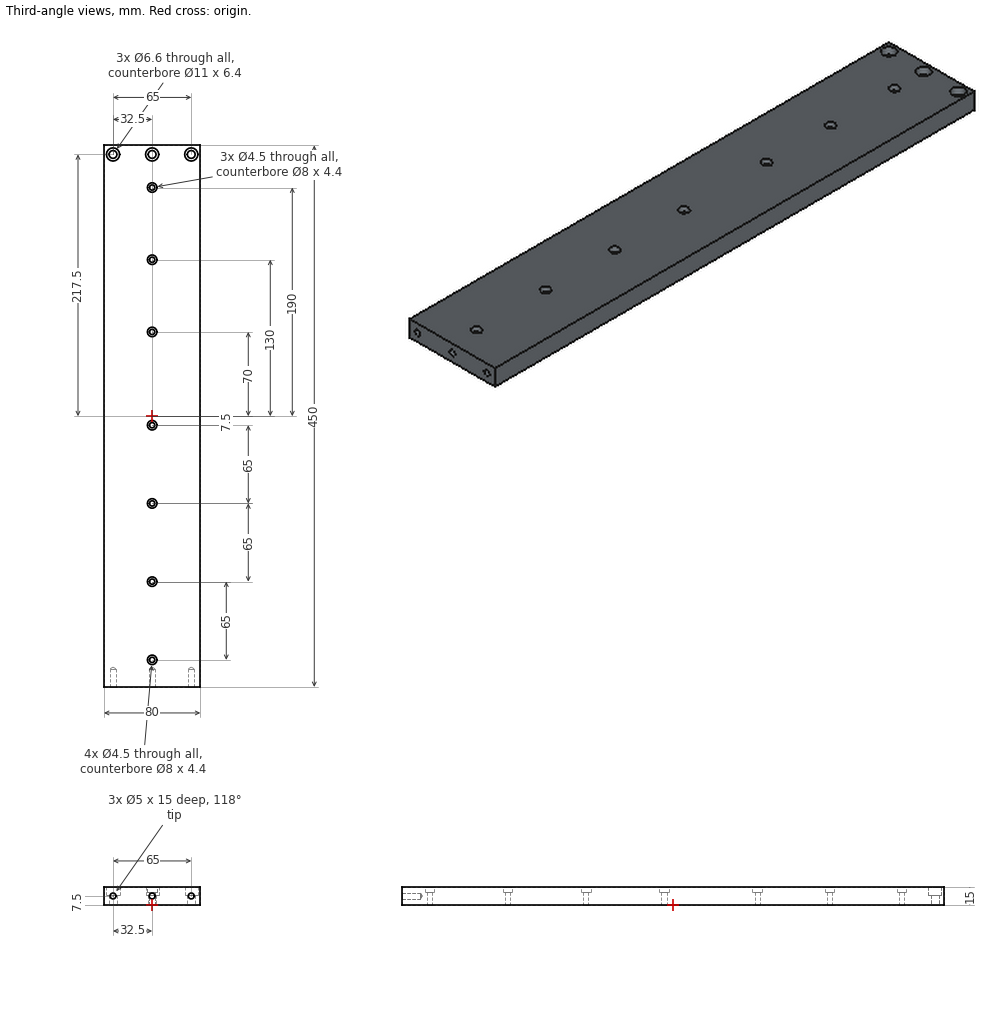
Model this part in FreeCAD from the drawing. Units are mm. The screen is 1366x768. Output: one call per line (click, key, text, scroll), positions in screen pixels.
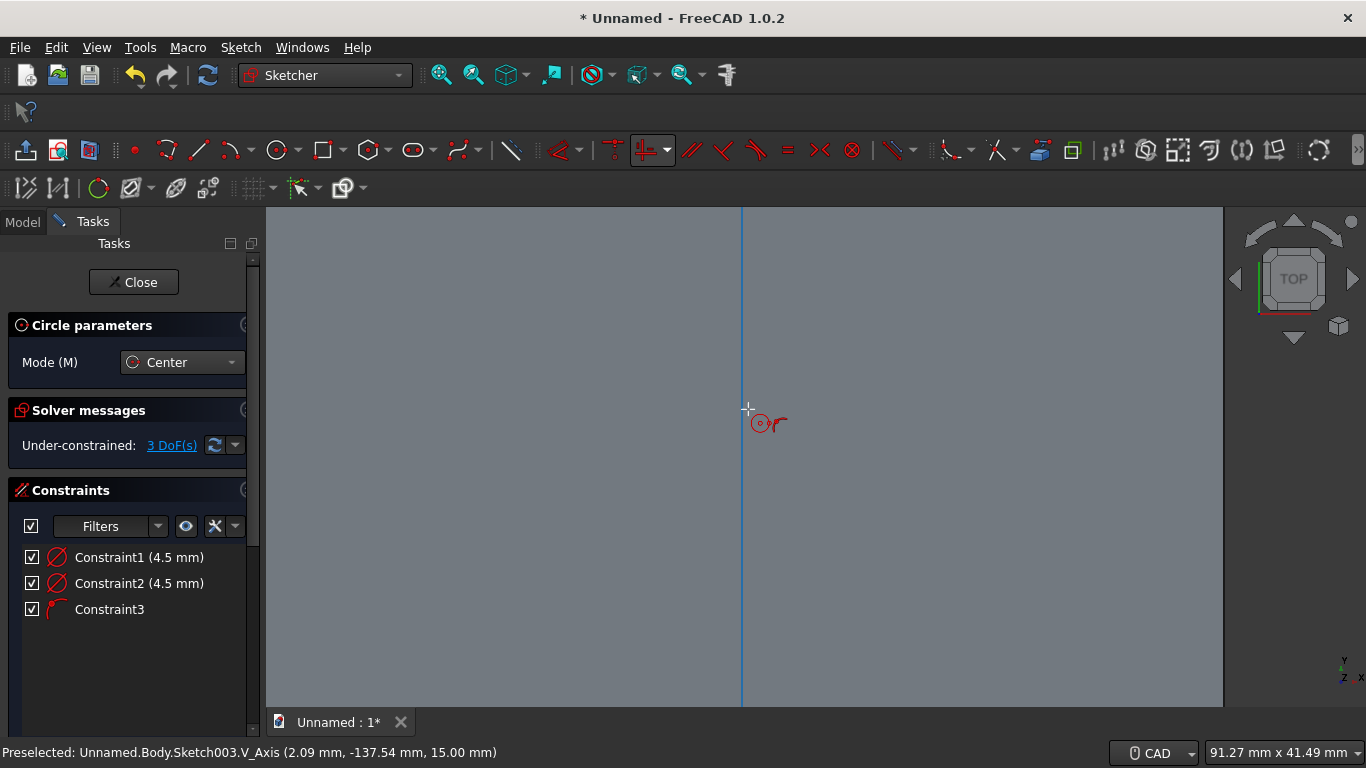
scroll(748, 409, down, 10)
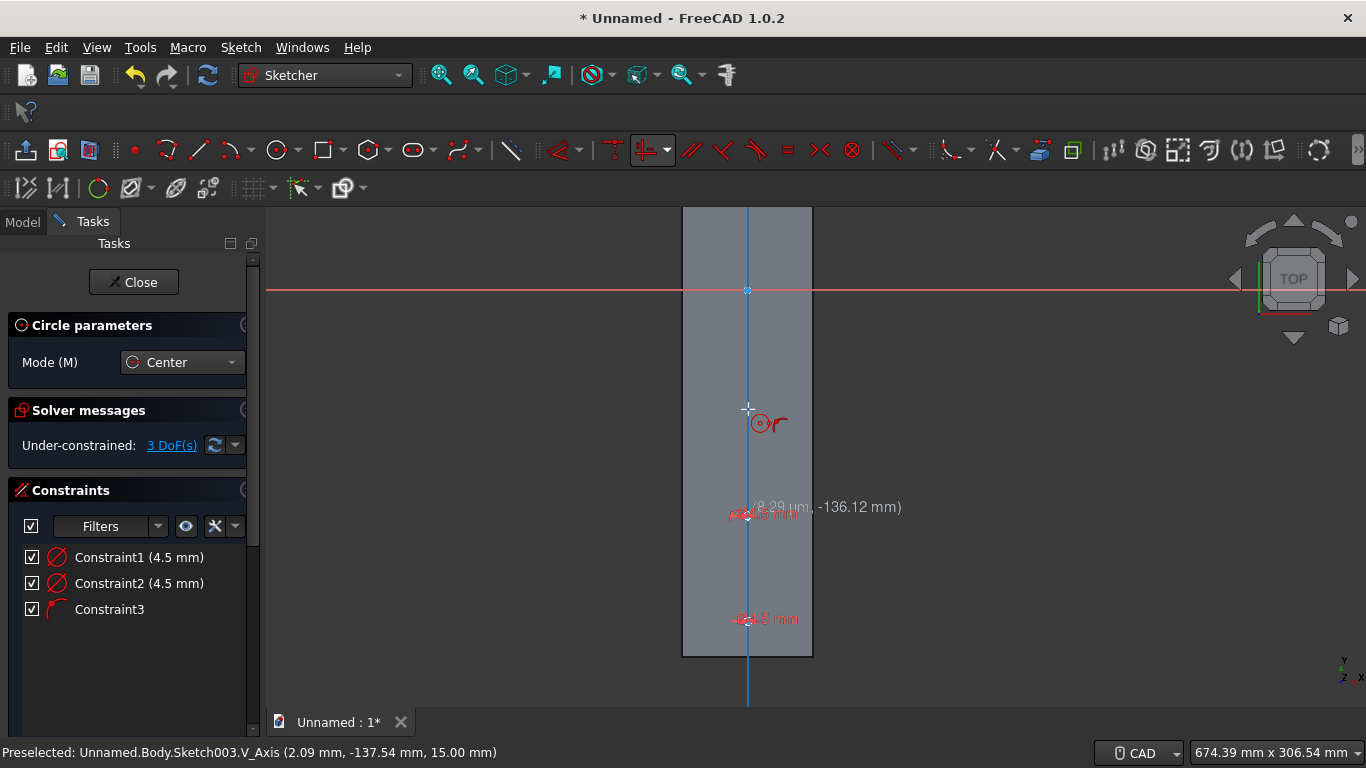
click(748, 409)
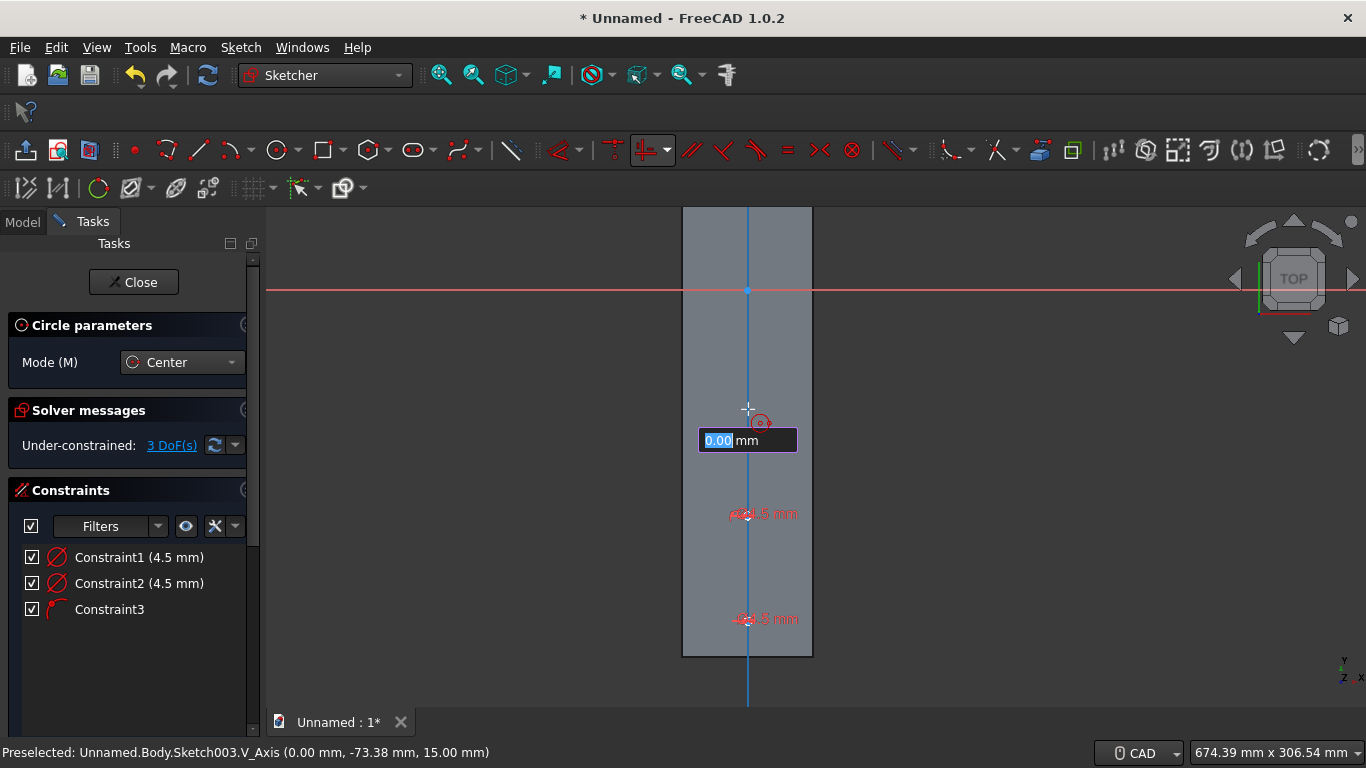
scroll(751, 407, up, 8)
move(750, 407)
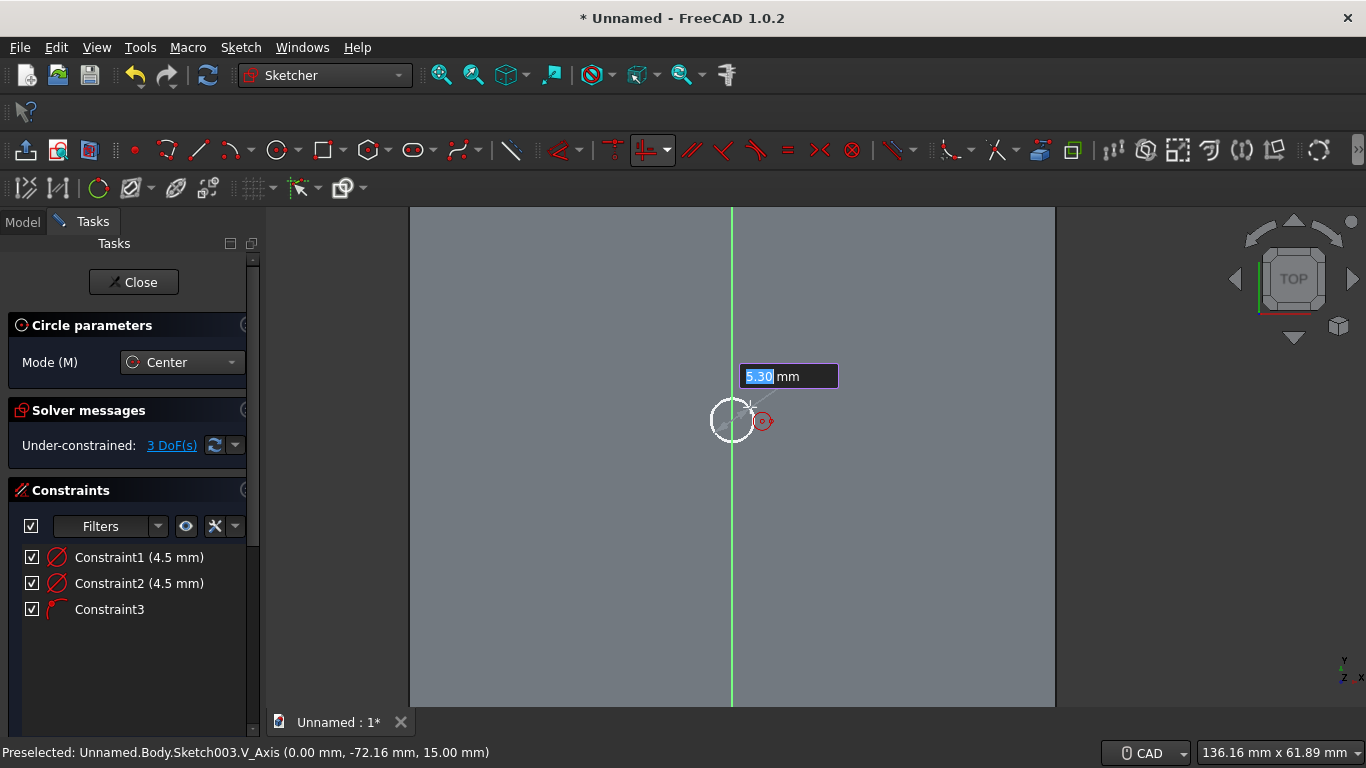
text(4.5)
key(Return)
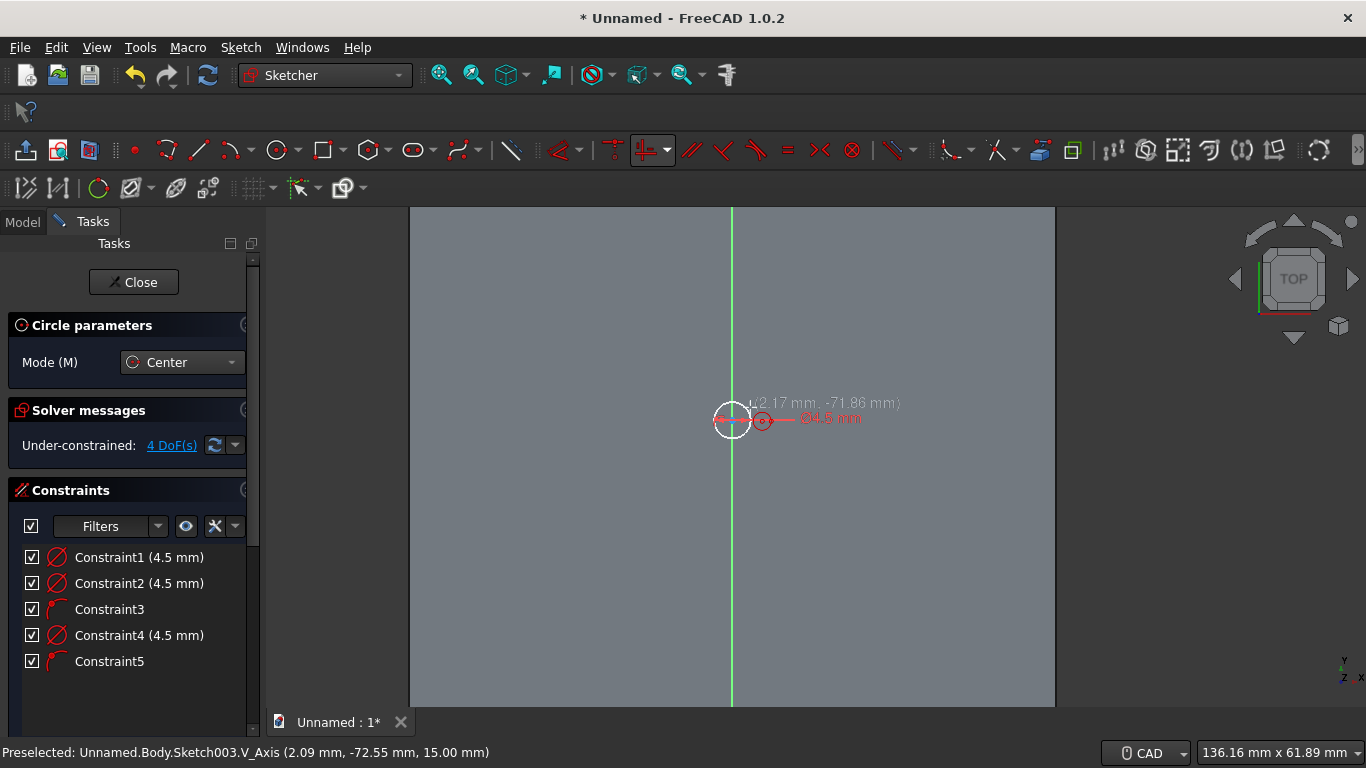
scroll(751, 407, down, 8)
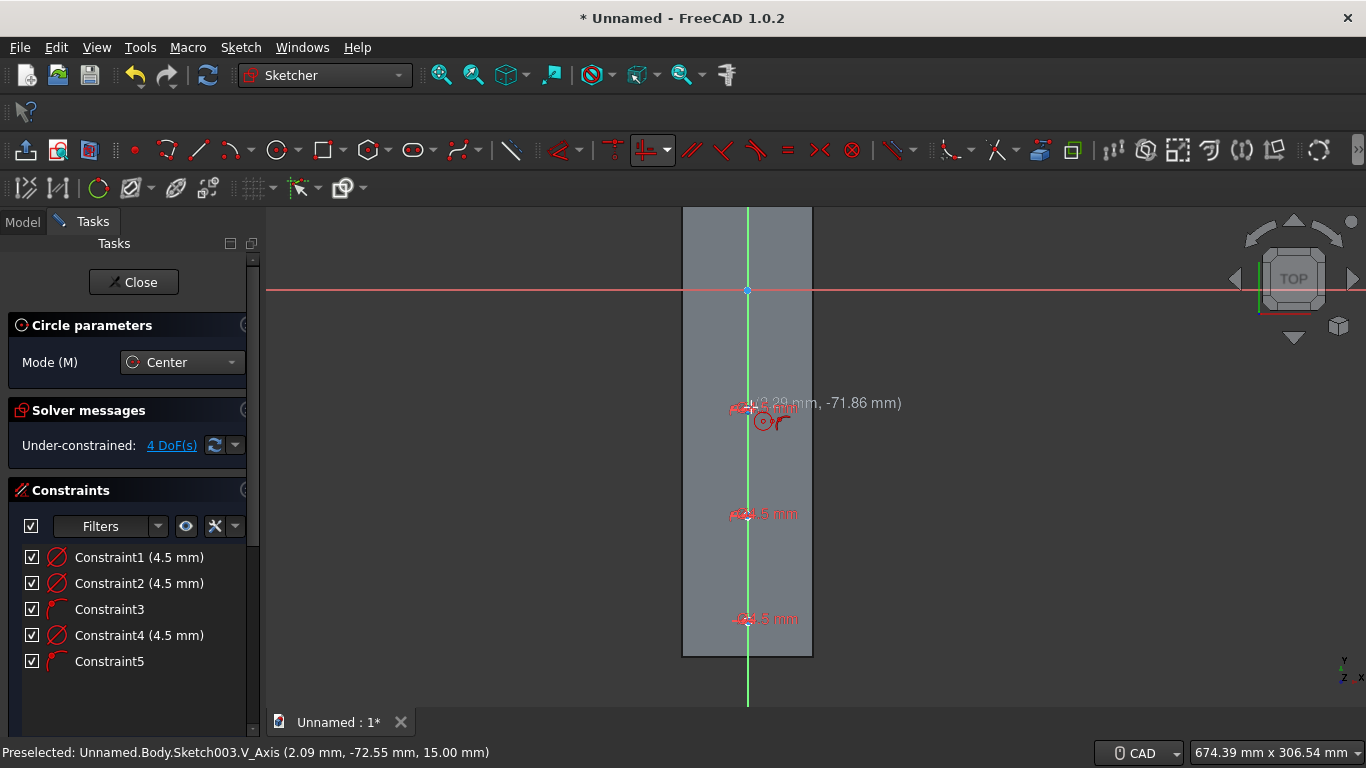
scroll(748, 303, up, 10)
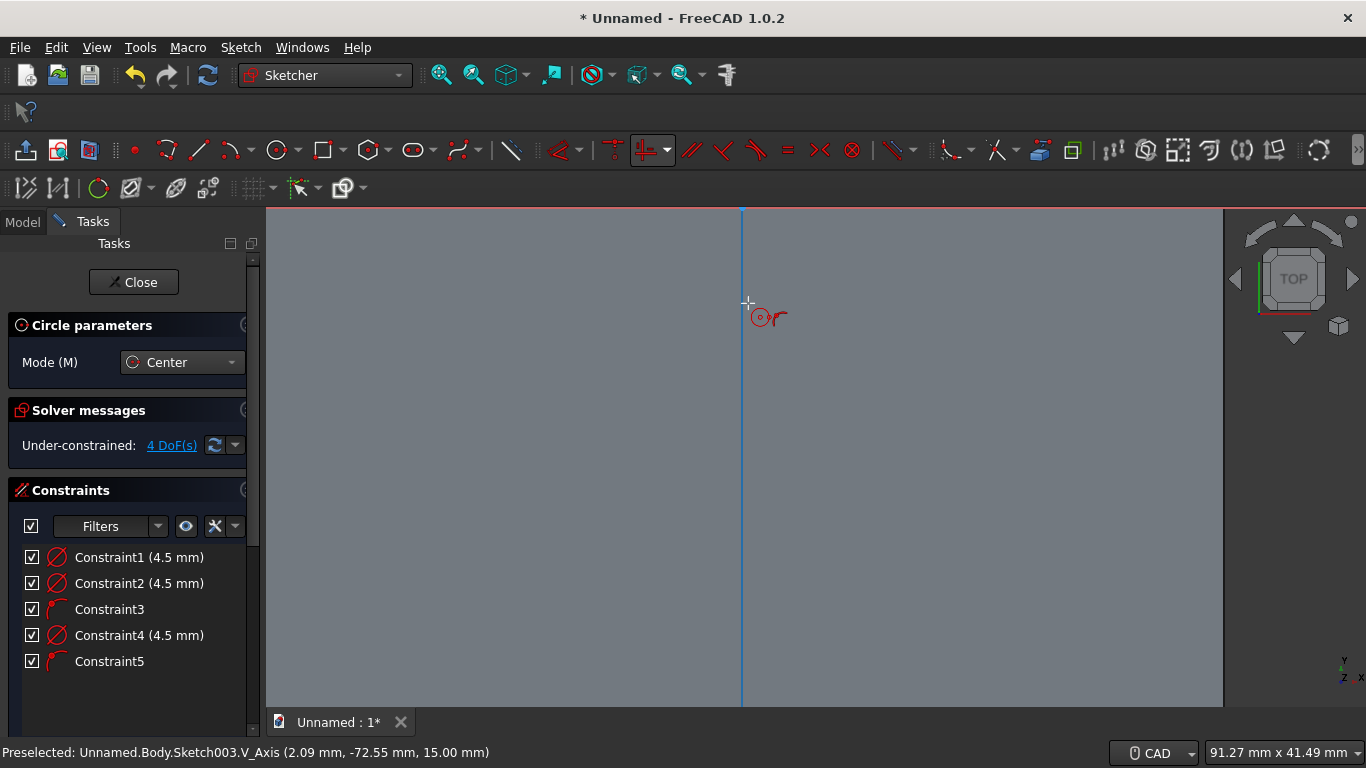
scroll(748, 303, down, 10)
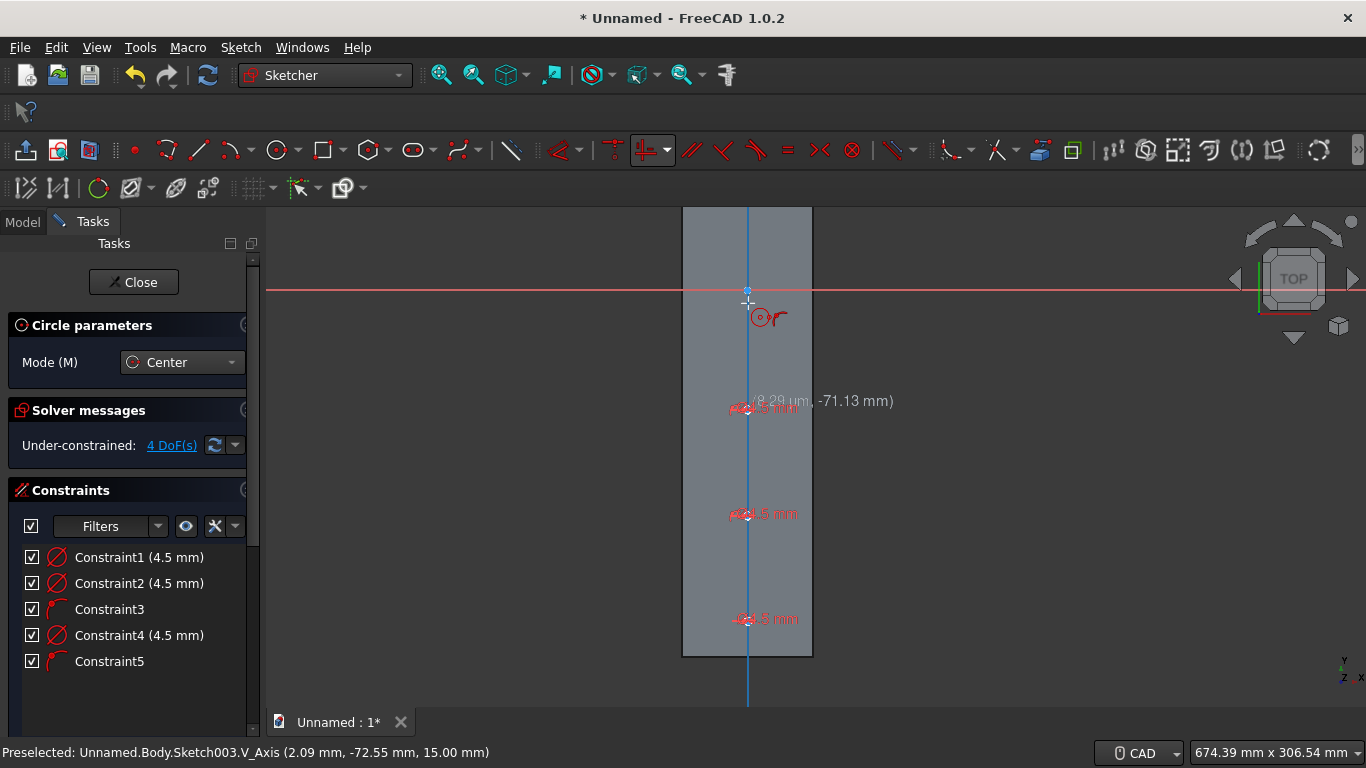
scroll(748, 303, up, 2)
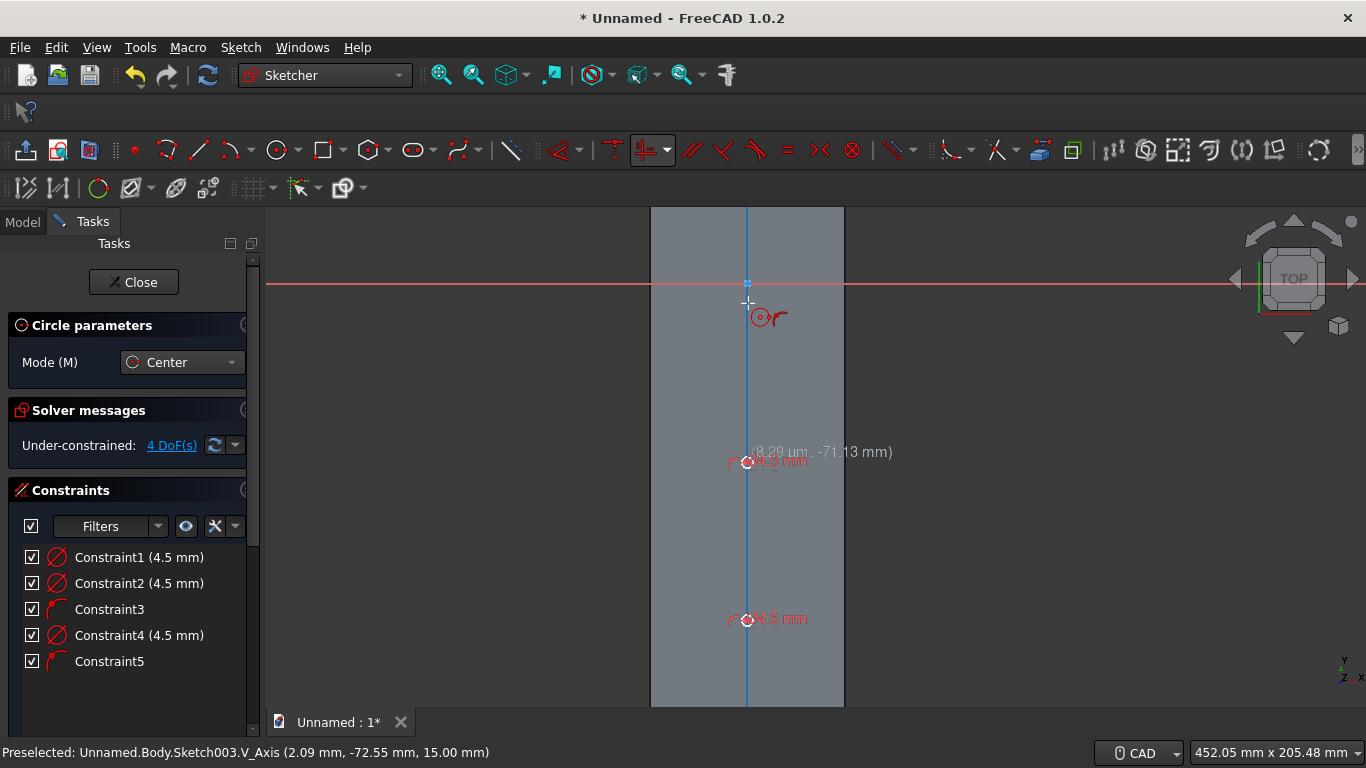
click(747, 302)